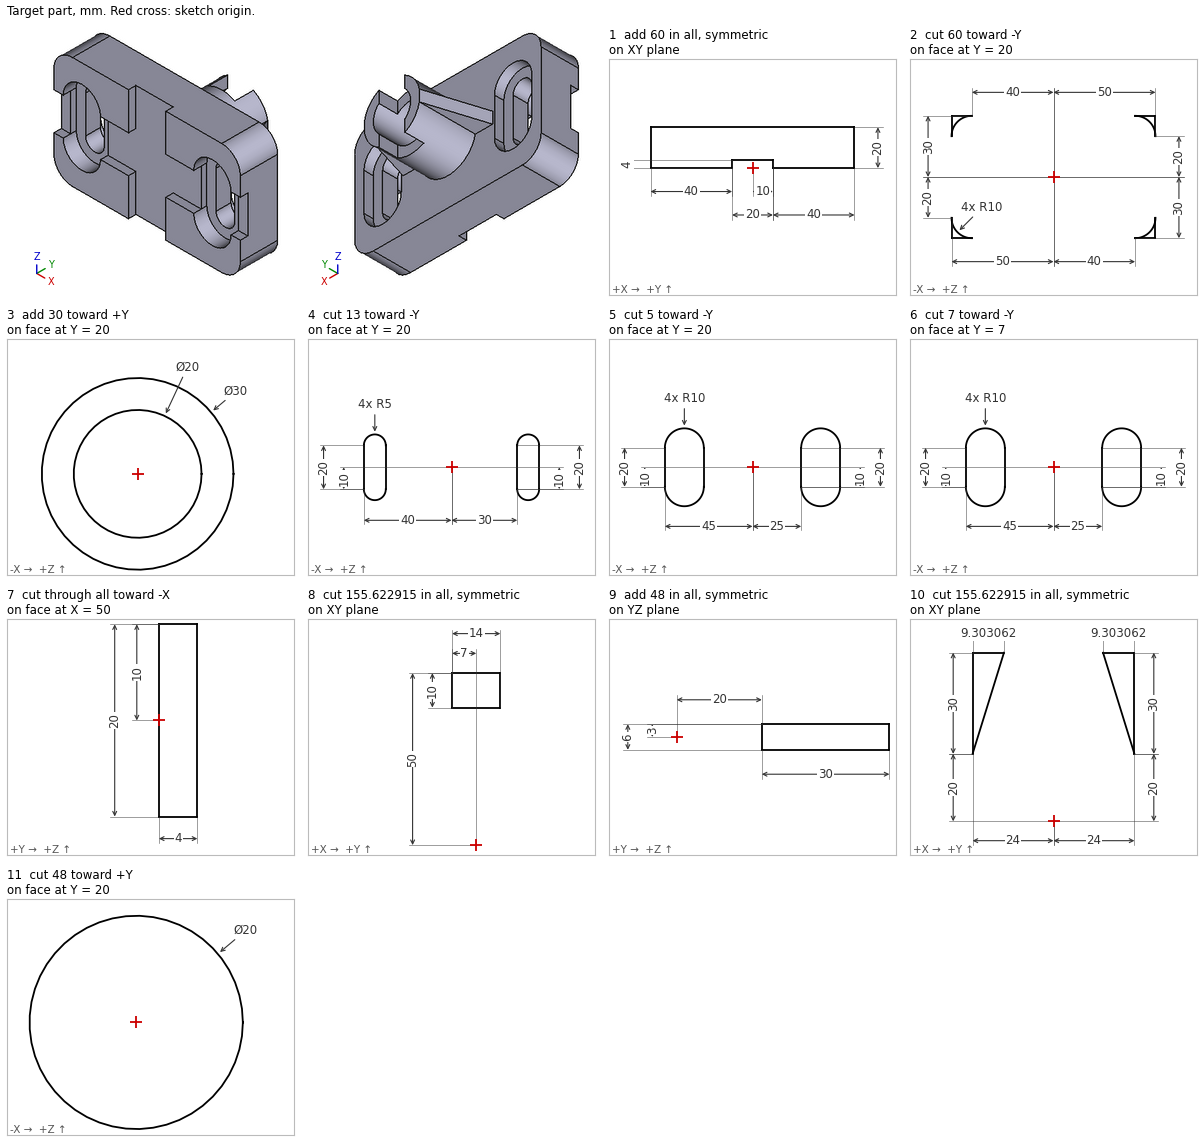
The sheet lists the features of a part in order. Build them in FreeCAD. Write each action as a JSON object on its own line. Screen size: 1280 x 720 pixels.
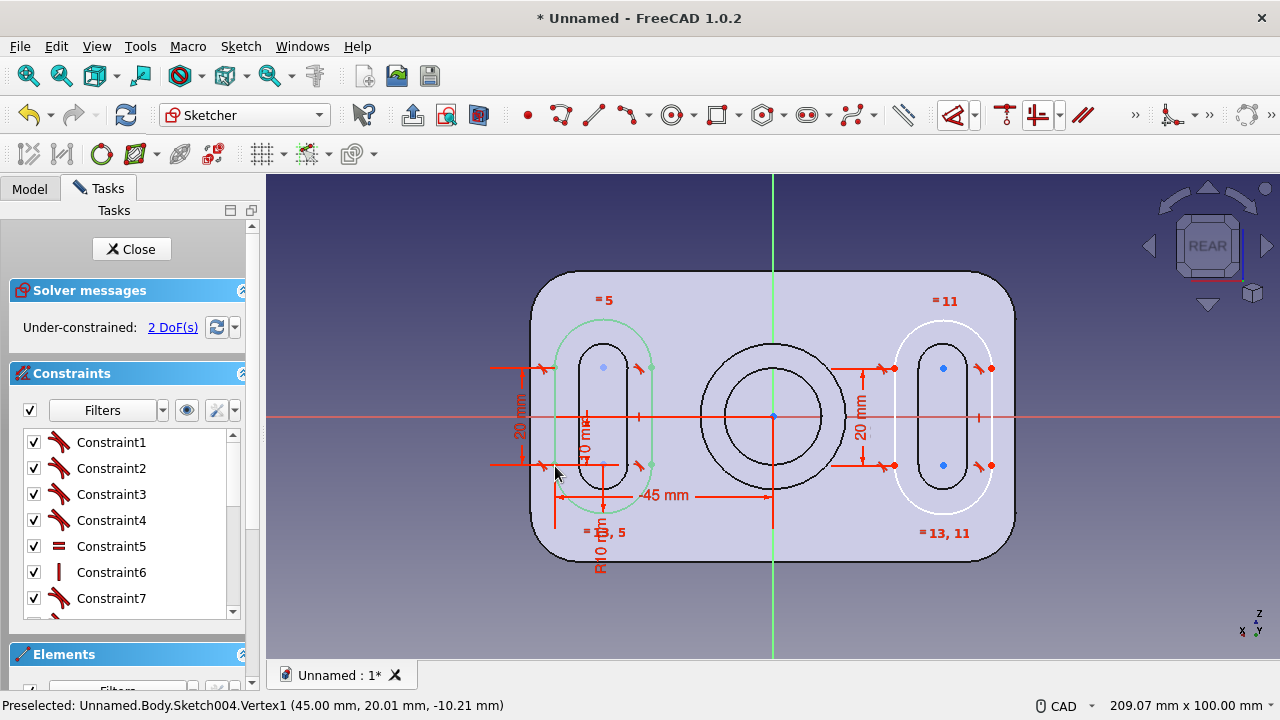
{"action": "left_click", "coordinate": [895, 466]}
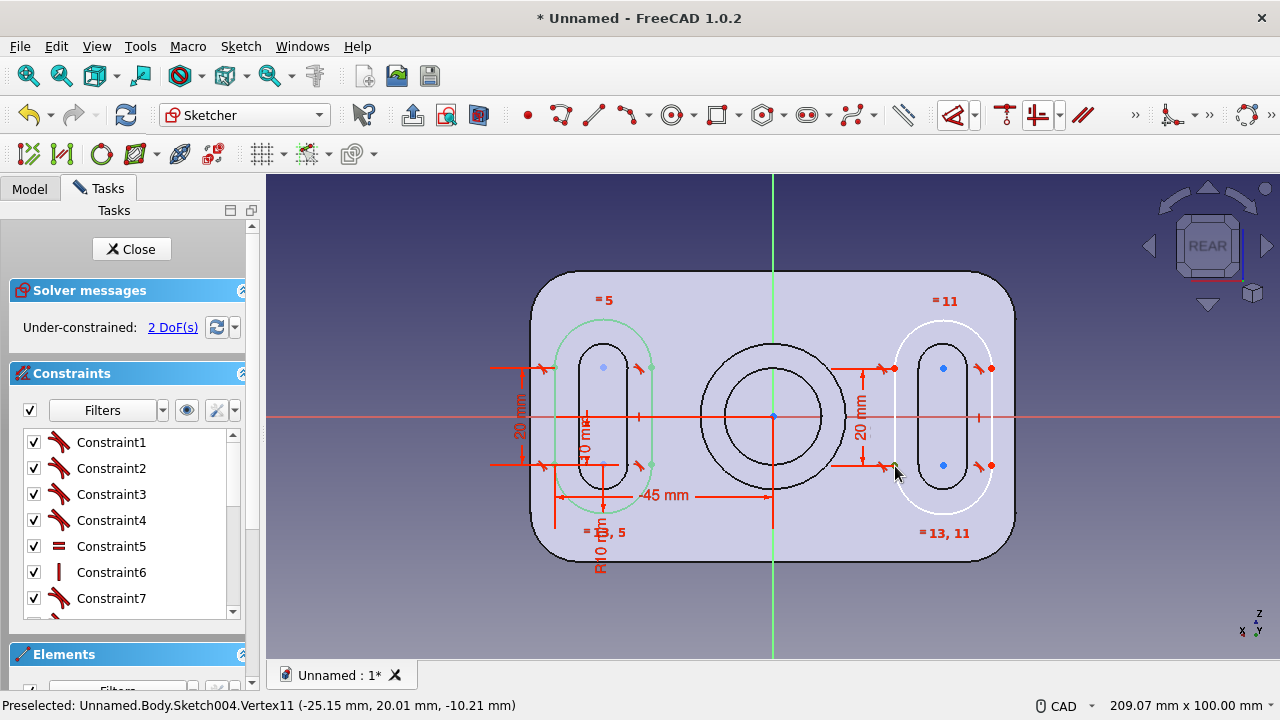
{"action": "key", "text": "l"}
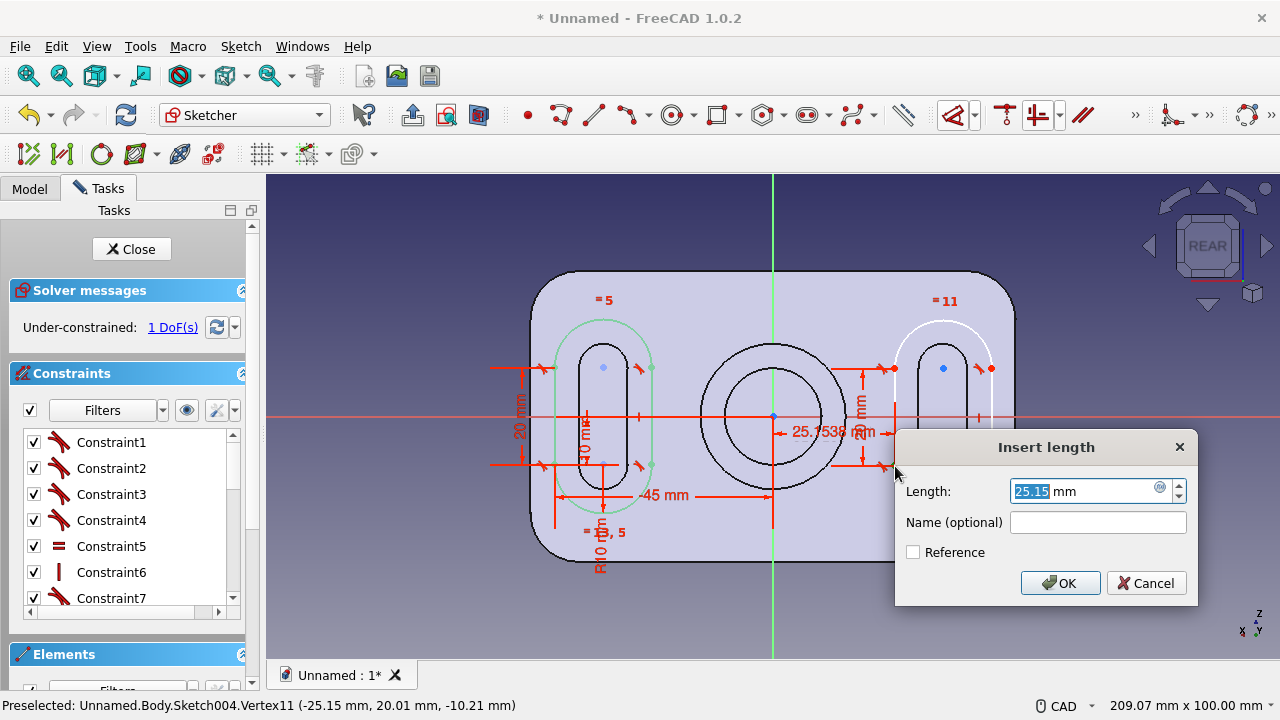
{"action": "type", "text": "25"}
{"action": "key", "text": "Return"}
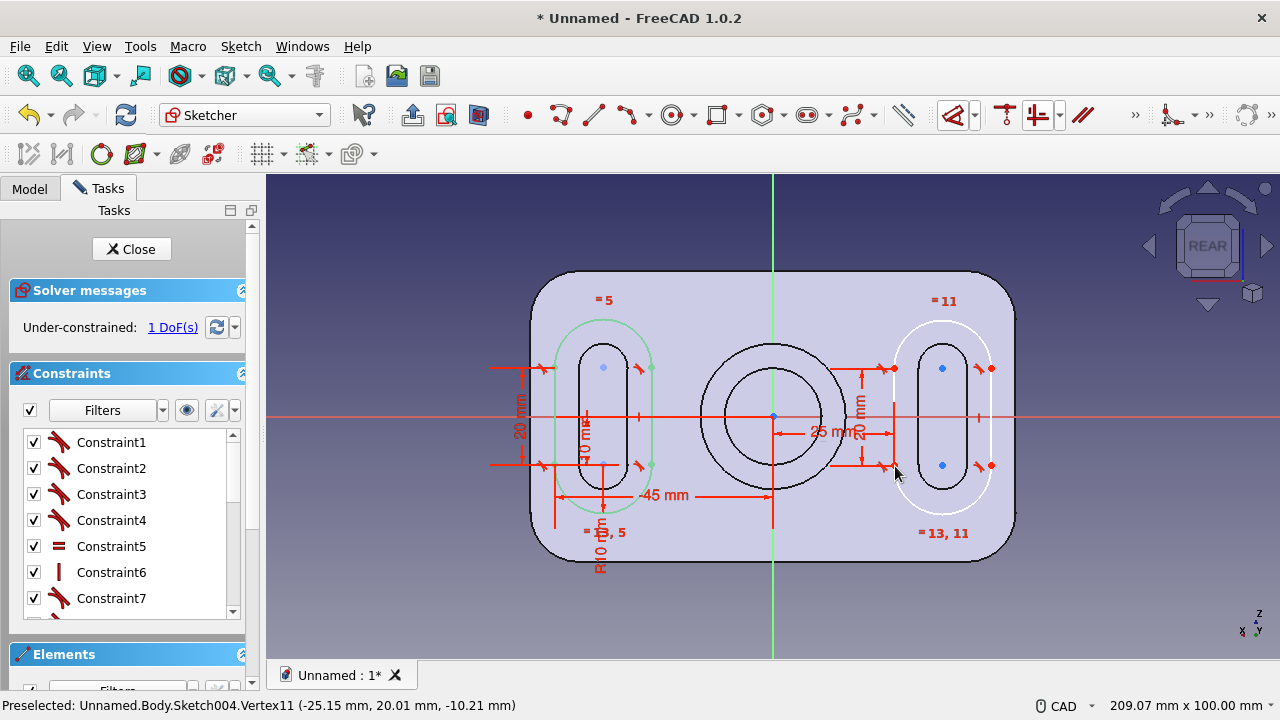
{"action": "left_click", "coordinate": [894, 466]}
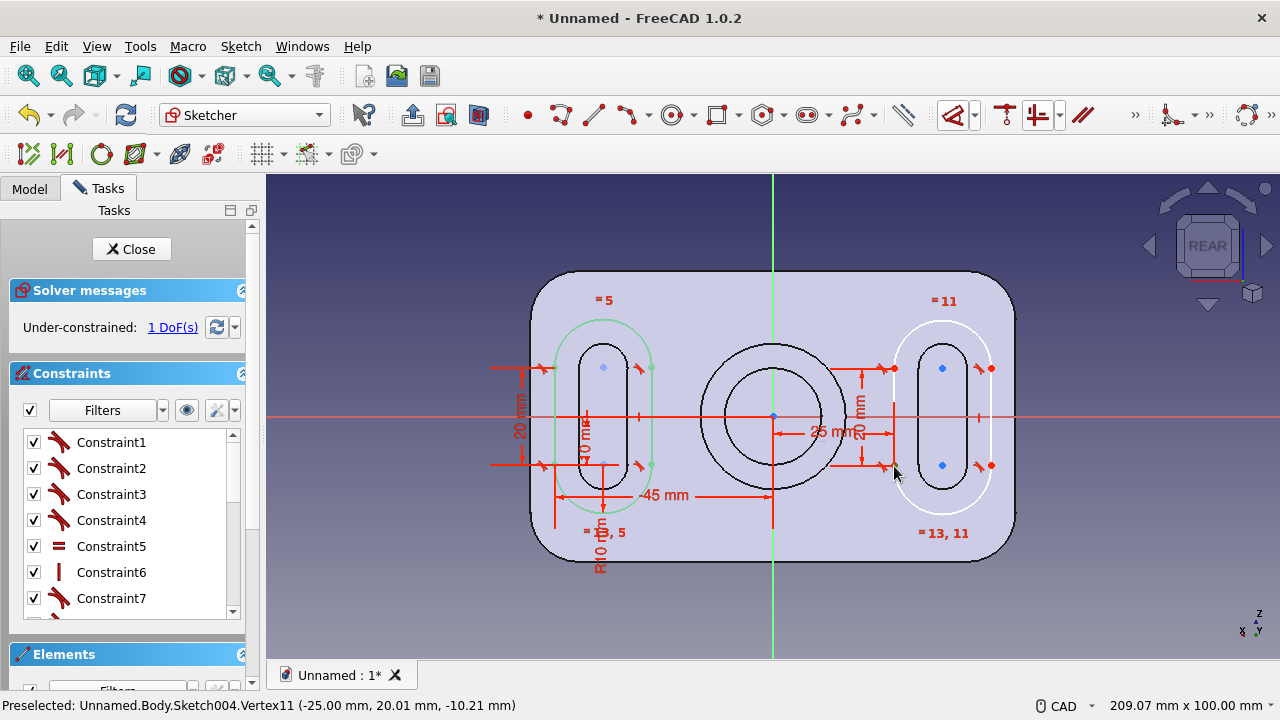
{"action": "key", "text": "i"}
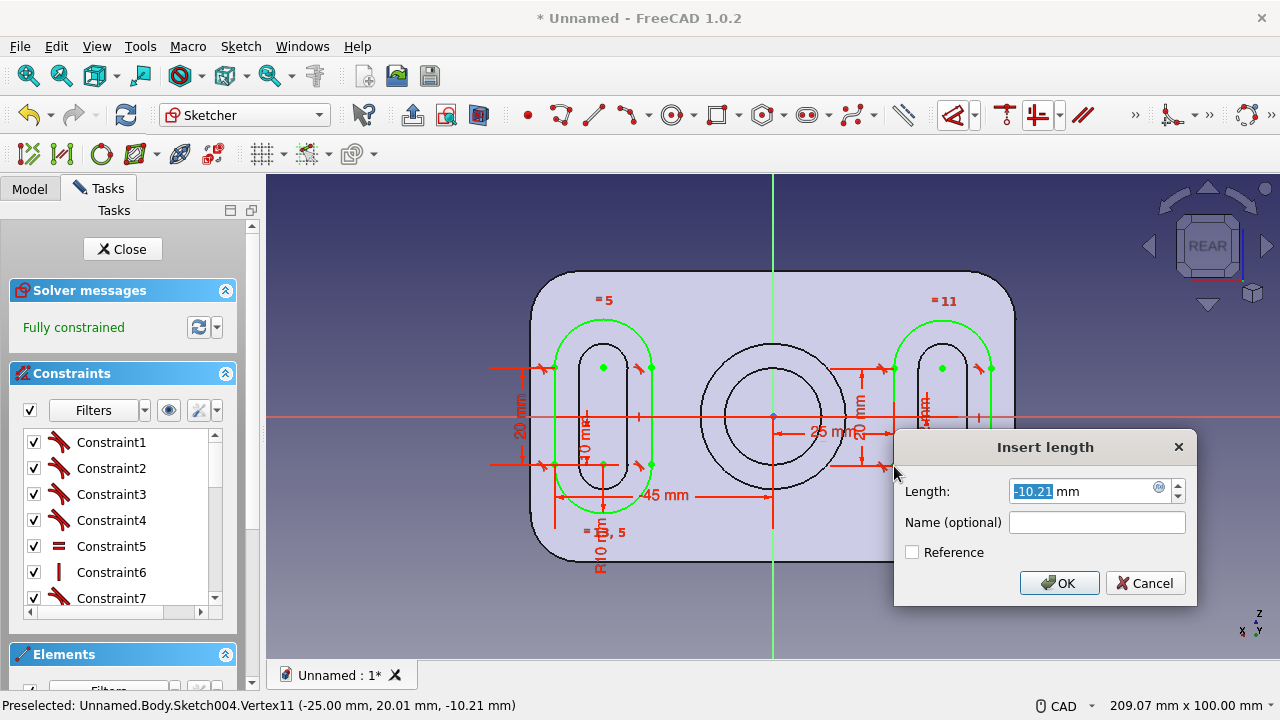
{"action": "type", "text": "-10"}
{"action": "key", "text": "Return"}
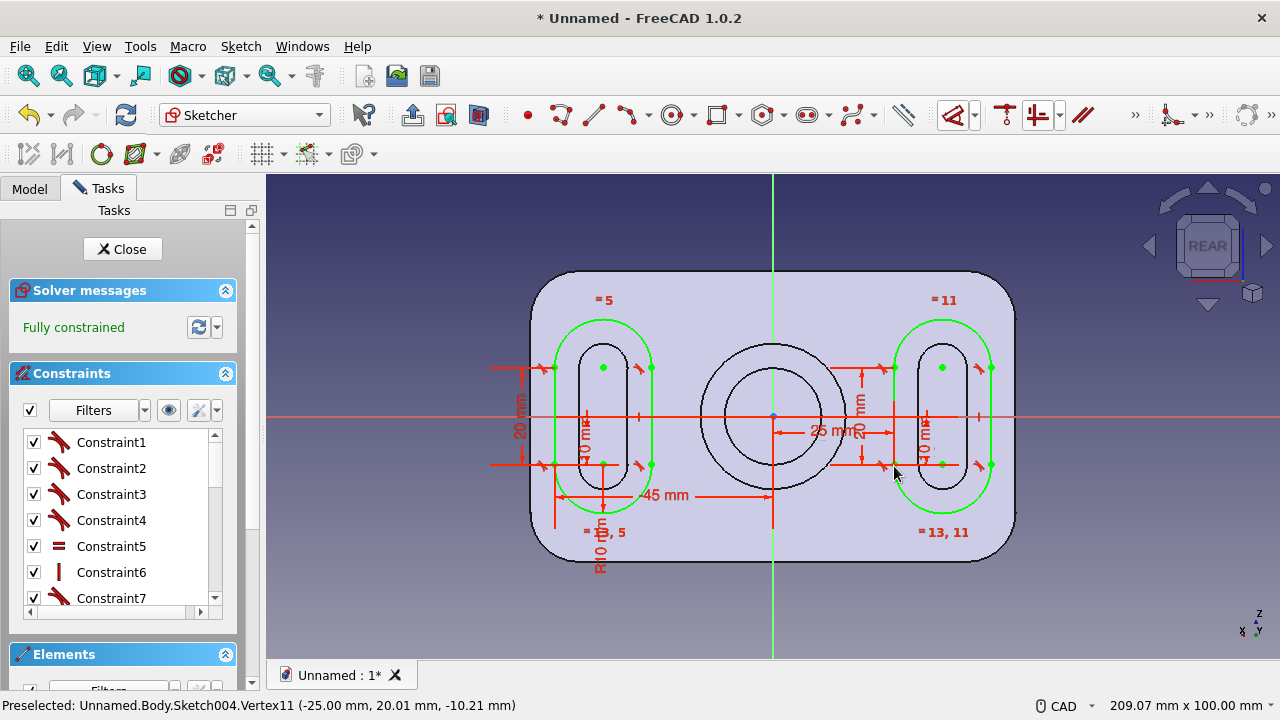
{"action": "left_click", "coordinate": [123, 249]}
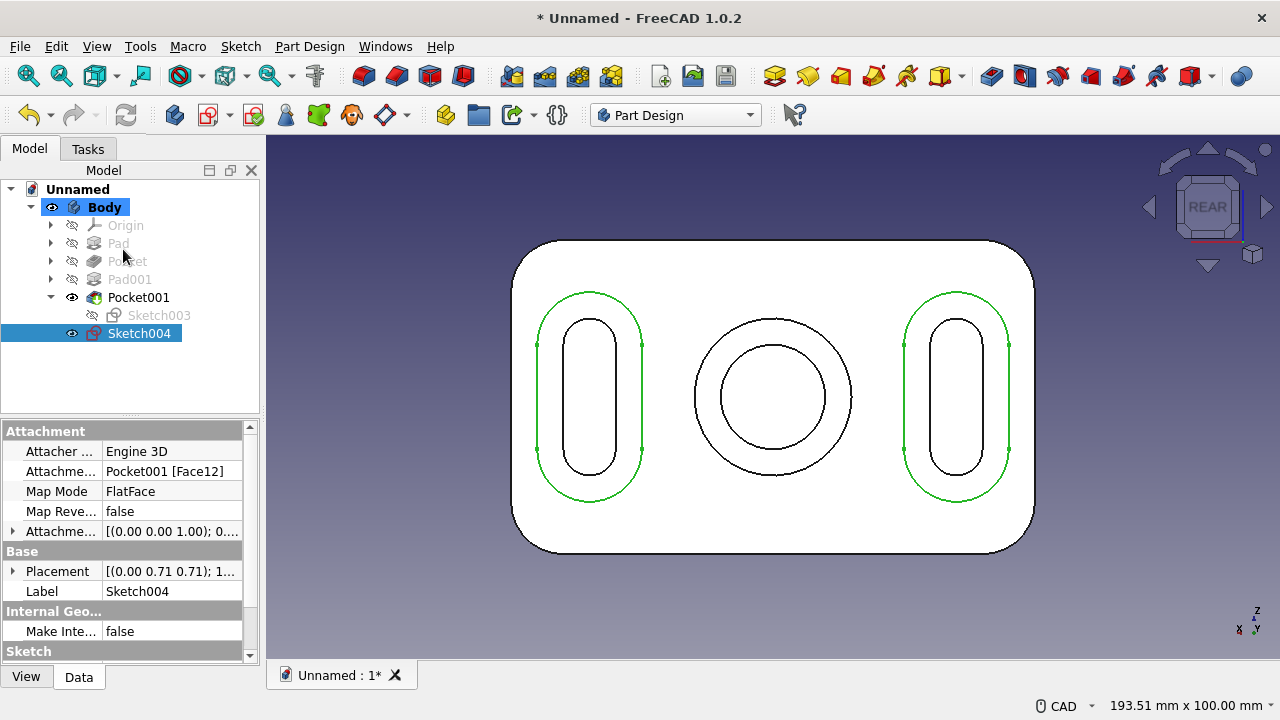
{"action": "left_click", "coordinate": [992, 76]}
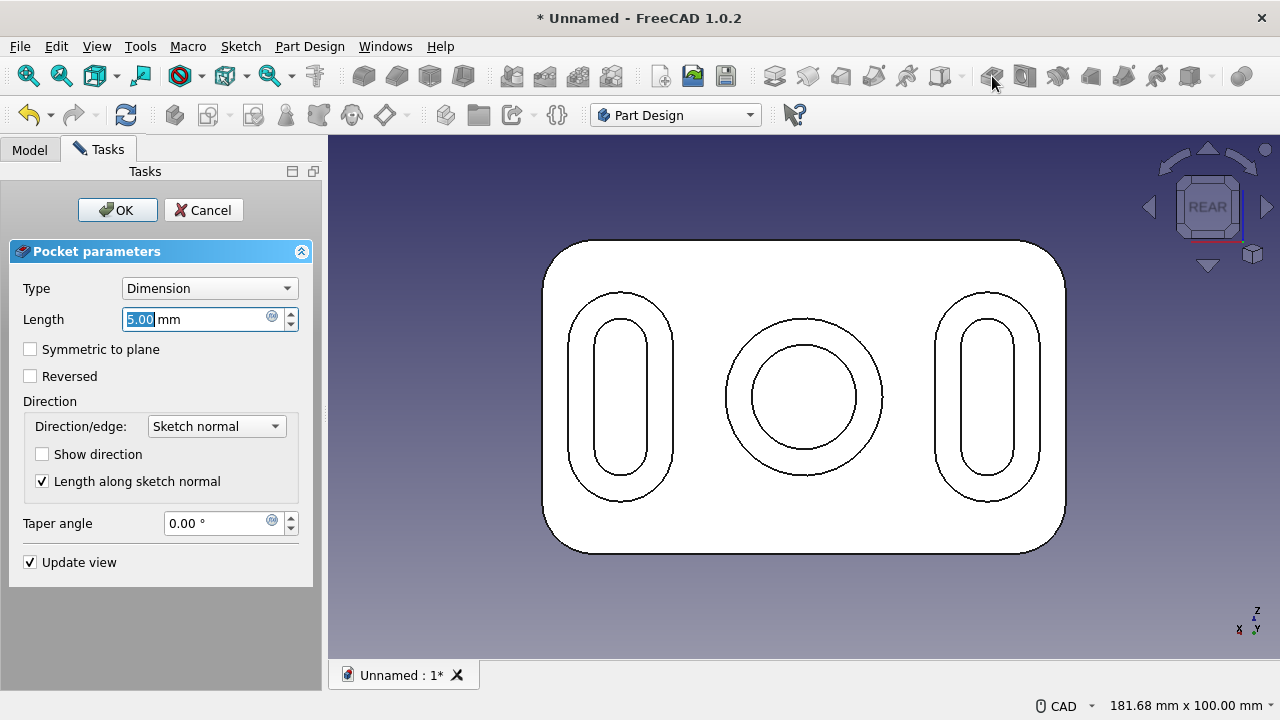
{"action": "type", "text": "5"}
{"action": "key", "text": "Tab"}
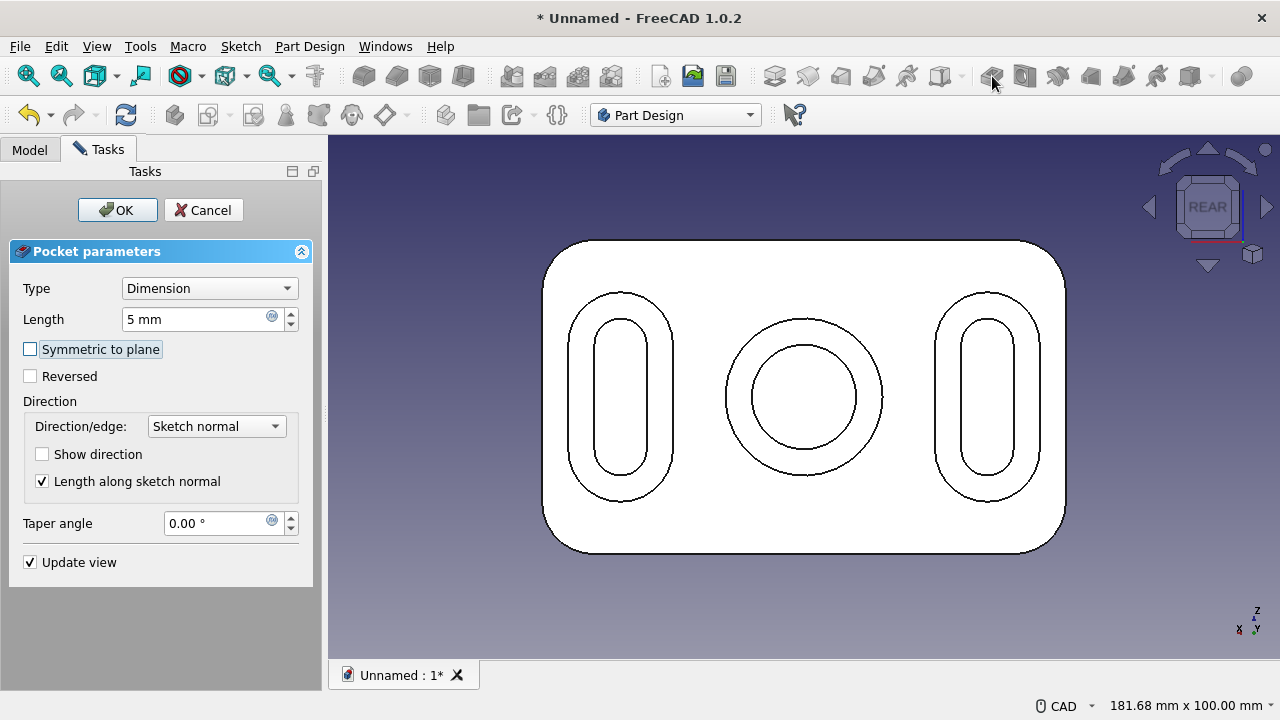
{"action": "left_click", "coordinate": [118, 210]}